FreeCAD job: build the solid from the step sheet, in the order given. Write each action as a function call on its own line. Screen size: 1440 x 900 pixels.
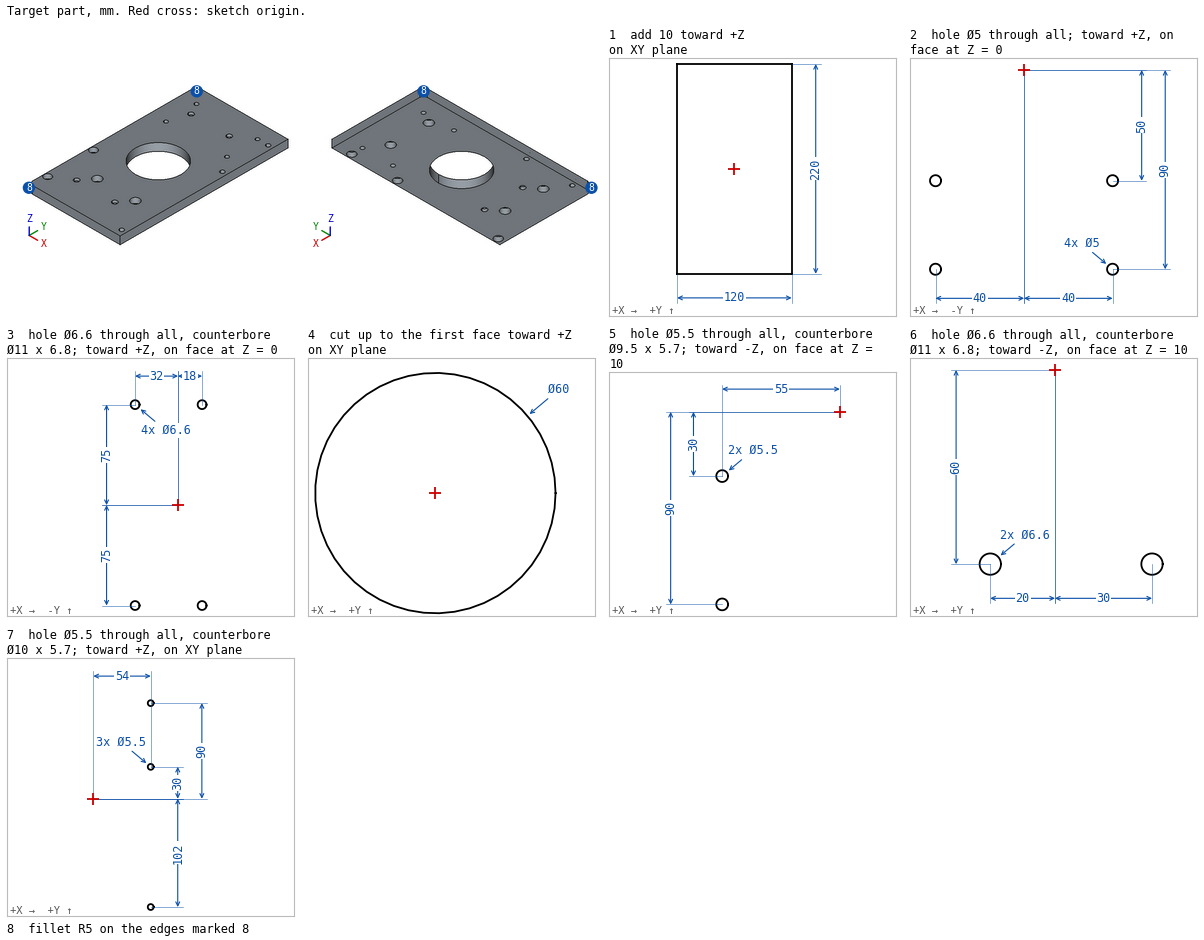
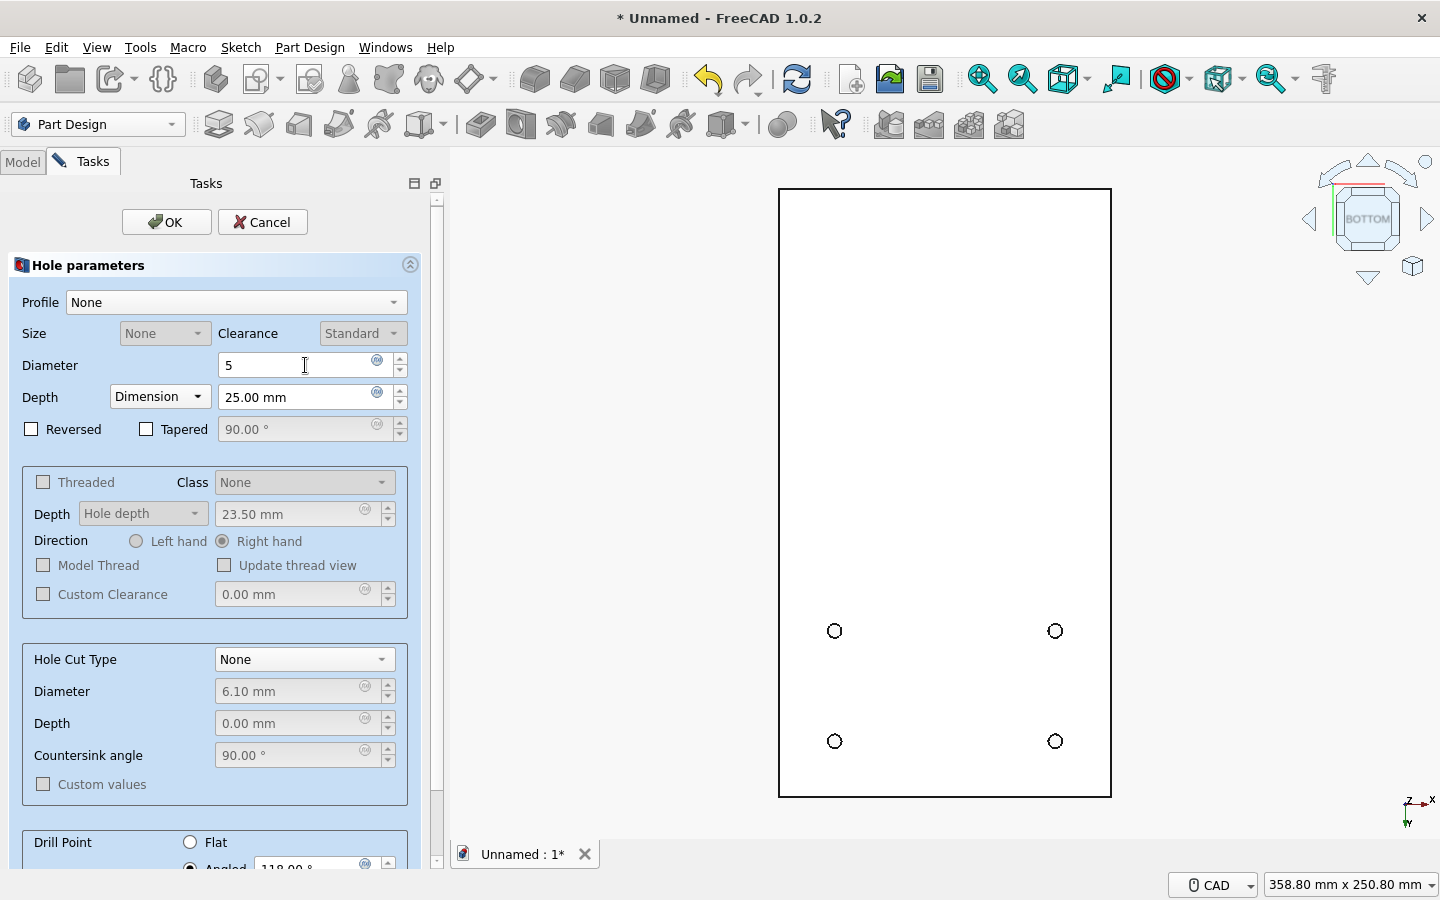
click(161, 396)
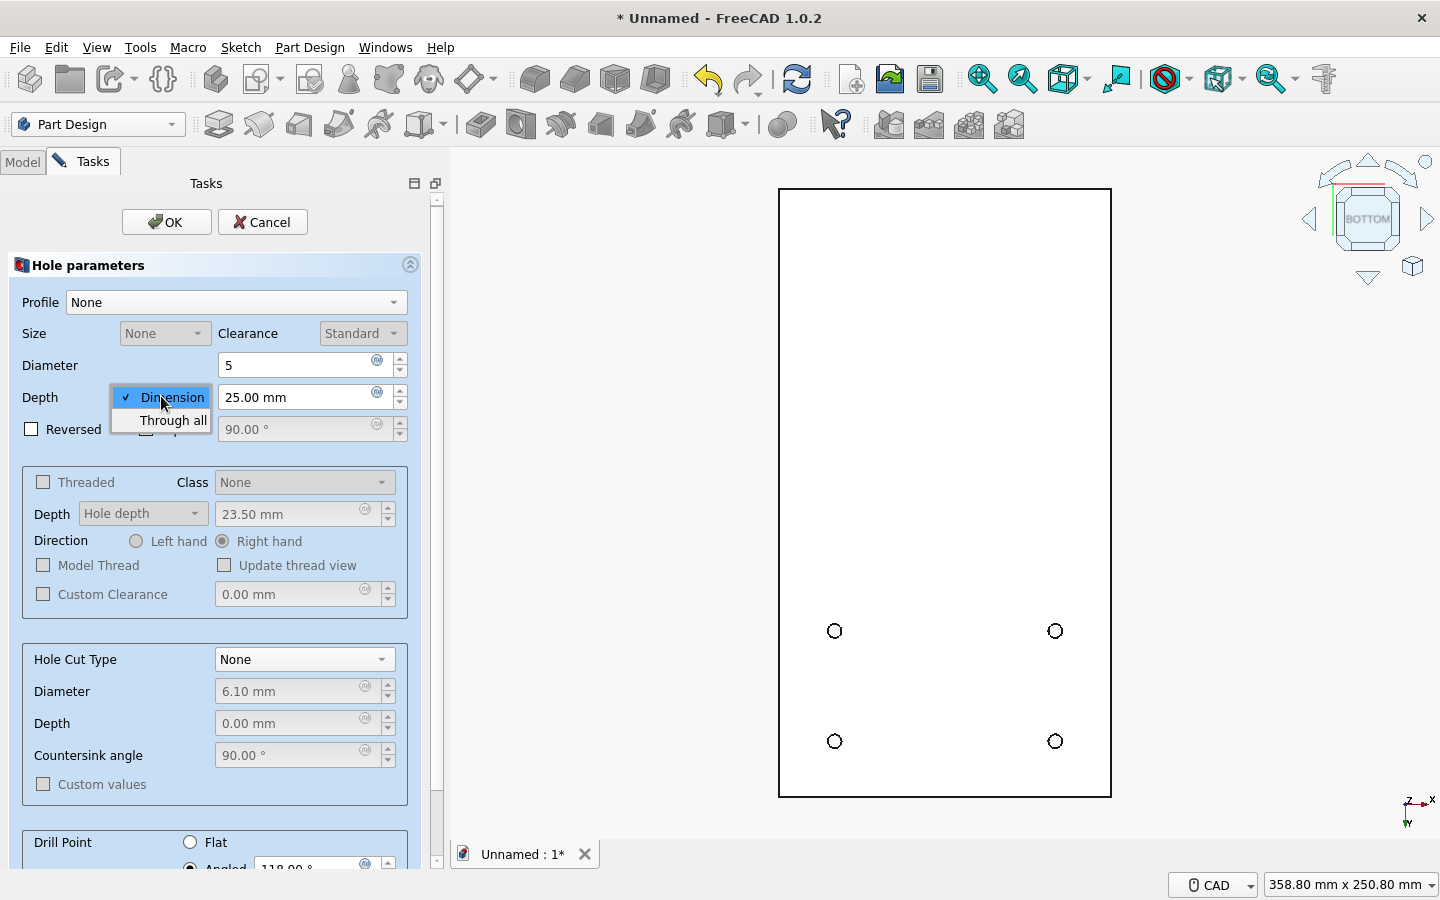
click(160, 420)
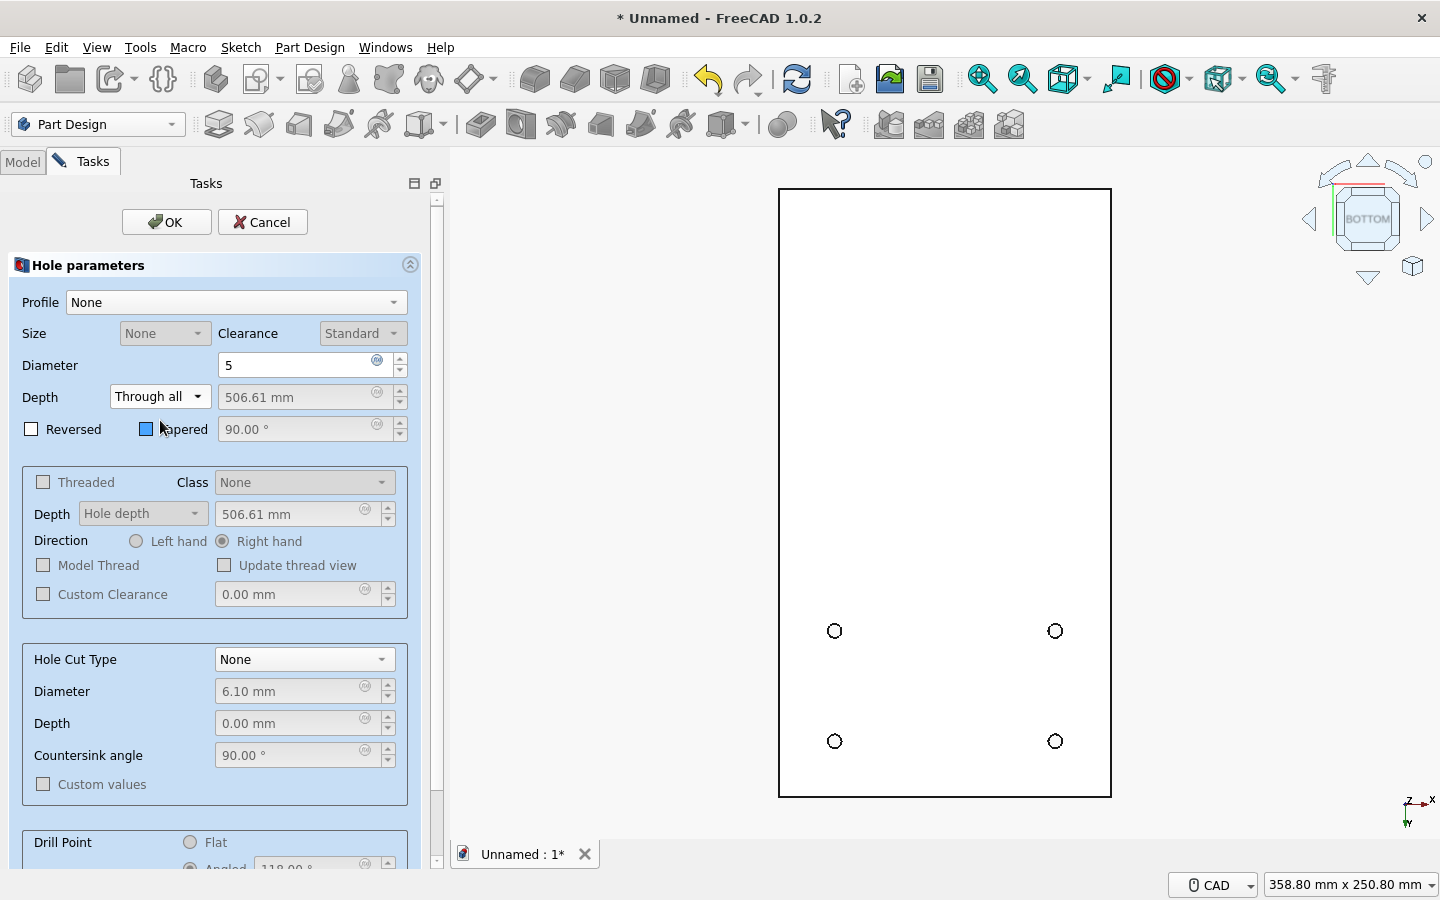
click(167, 222)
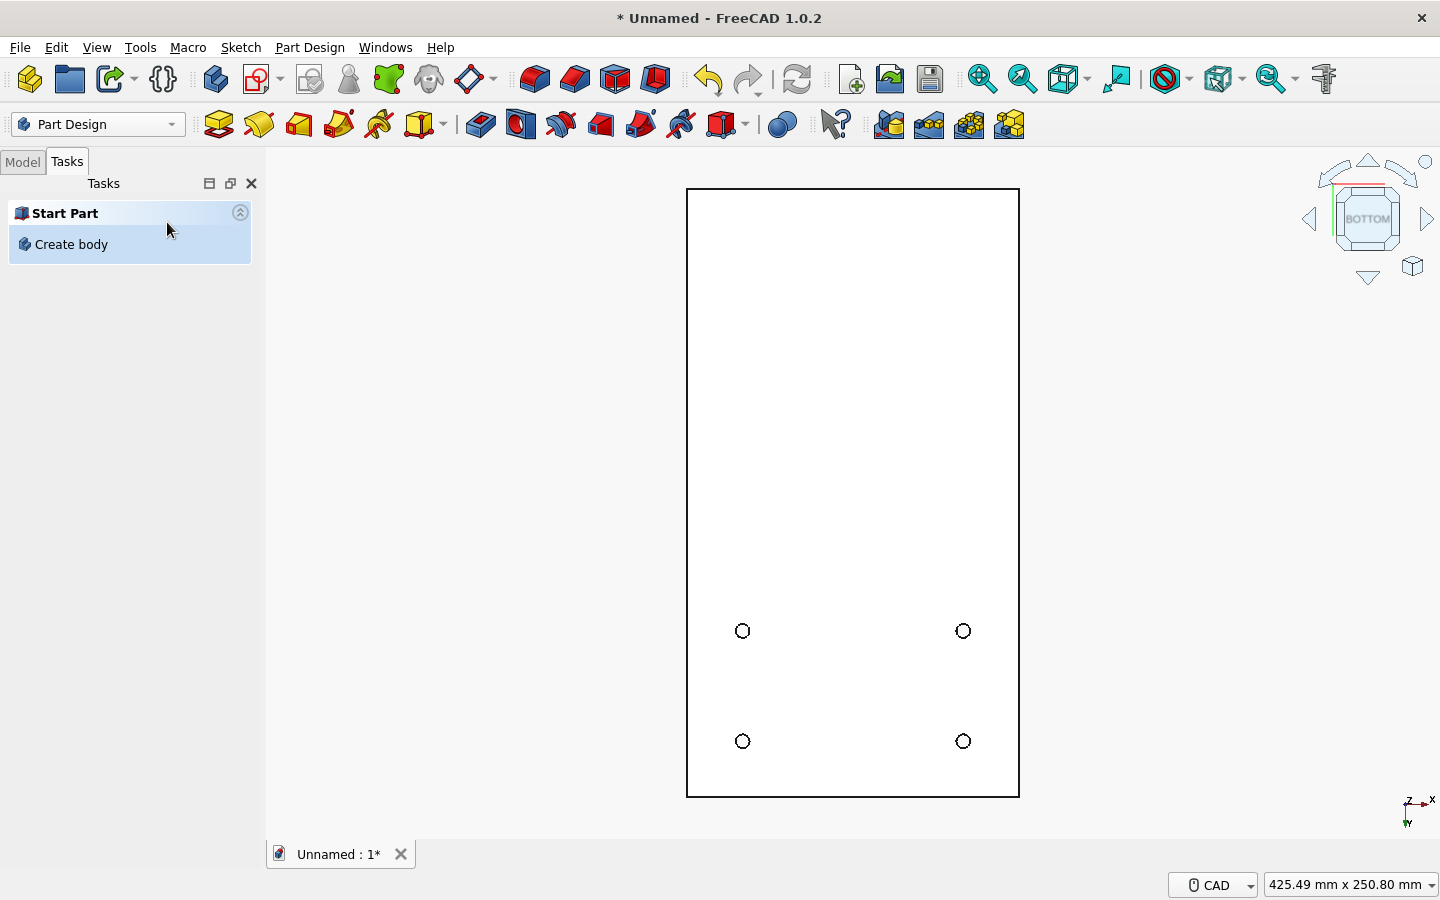
click(853, 492)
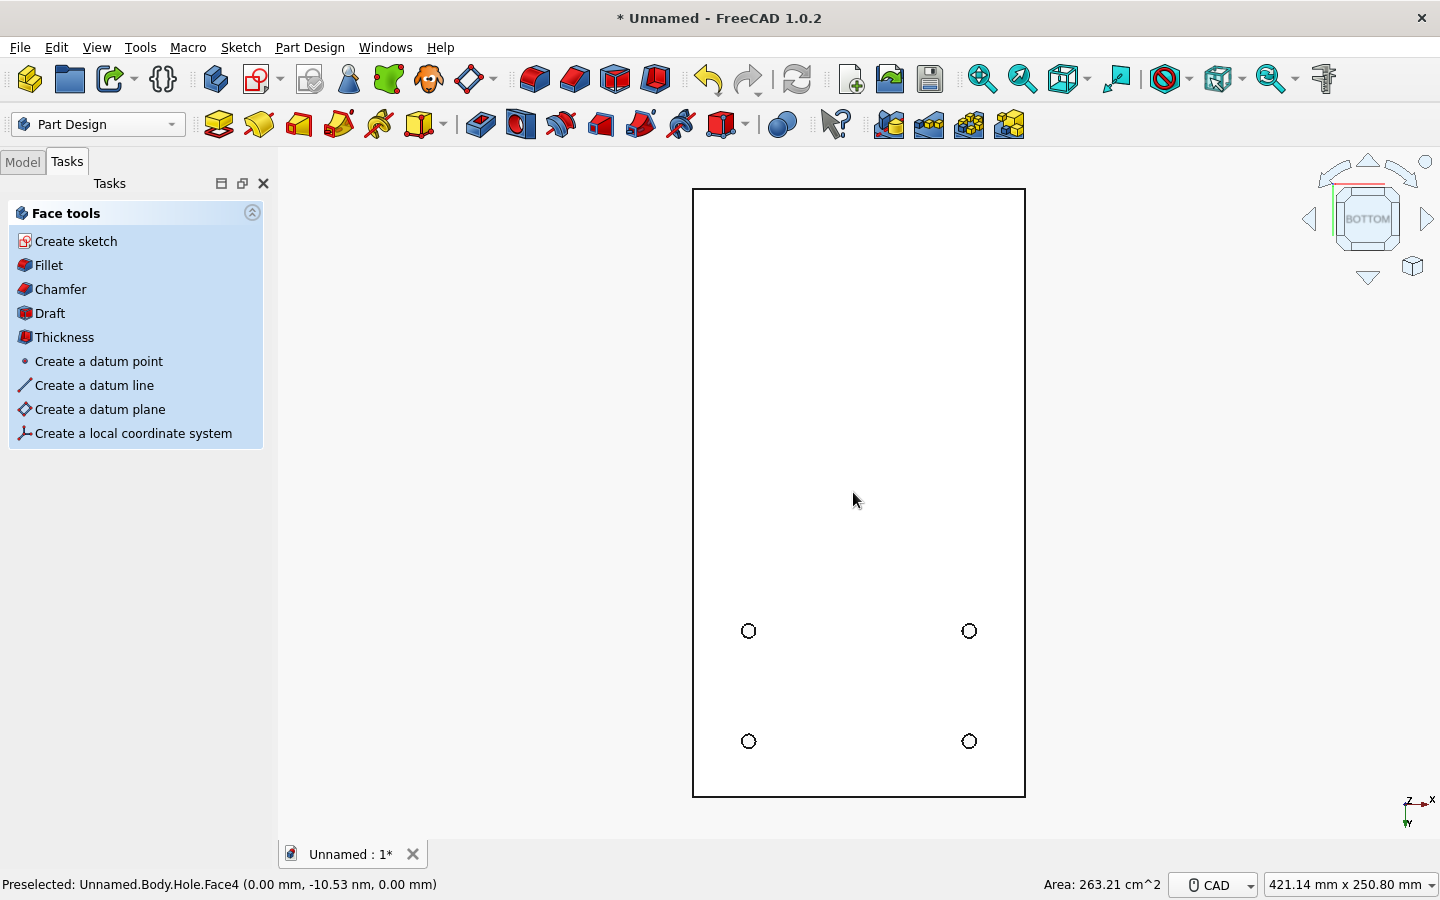
click(256, 80)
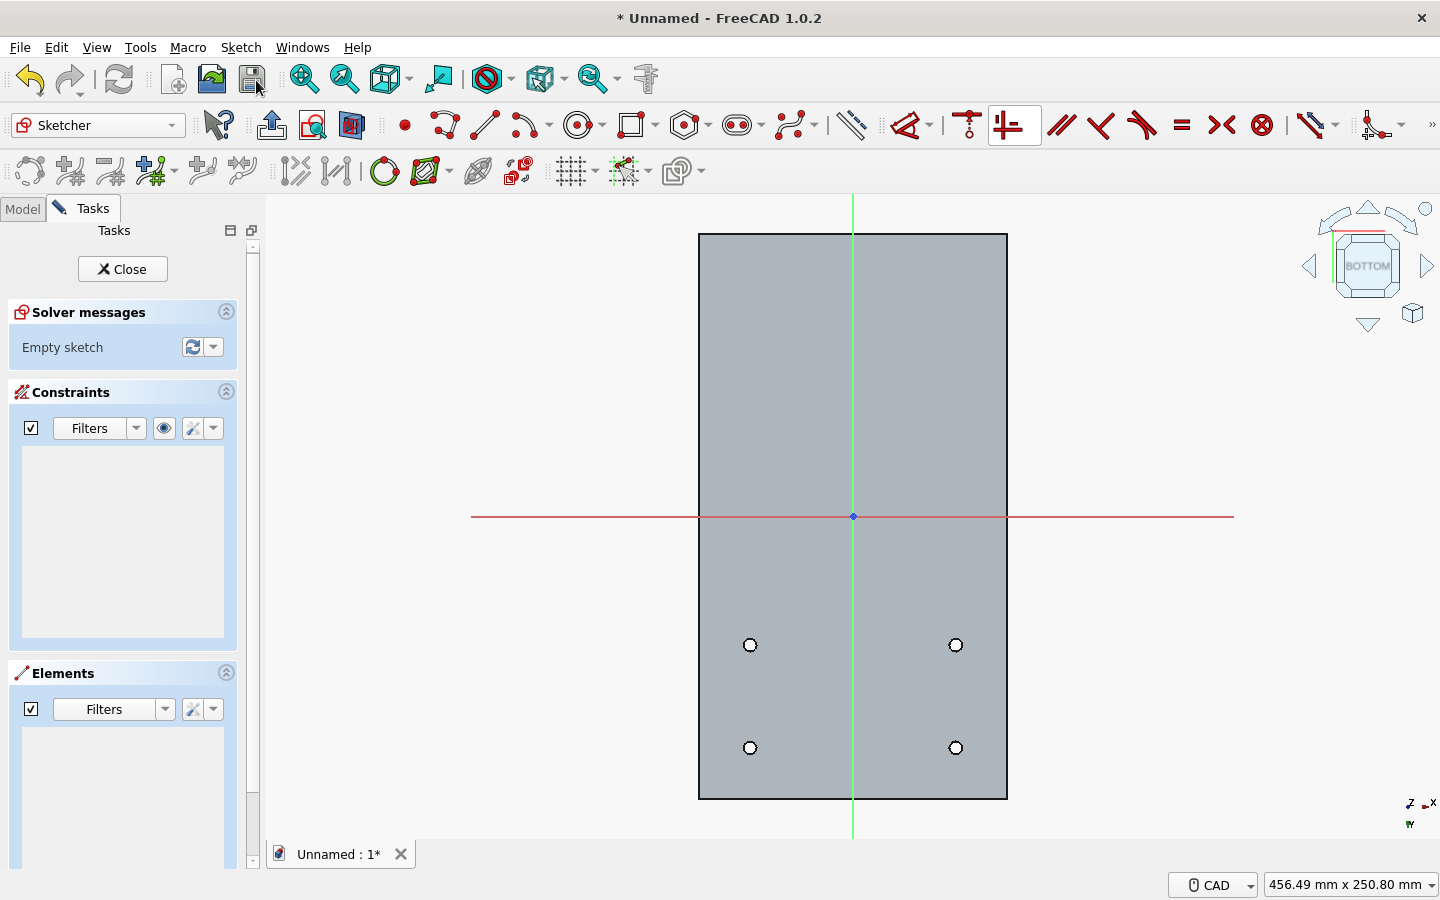
key(g)
key(c)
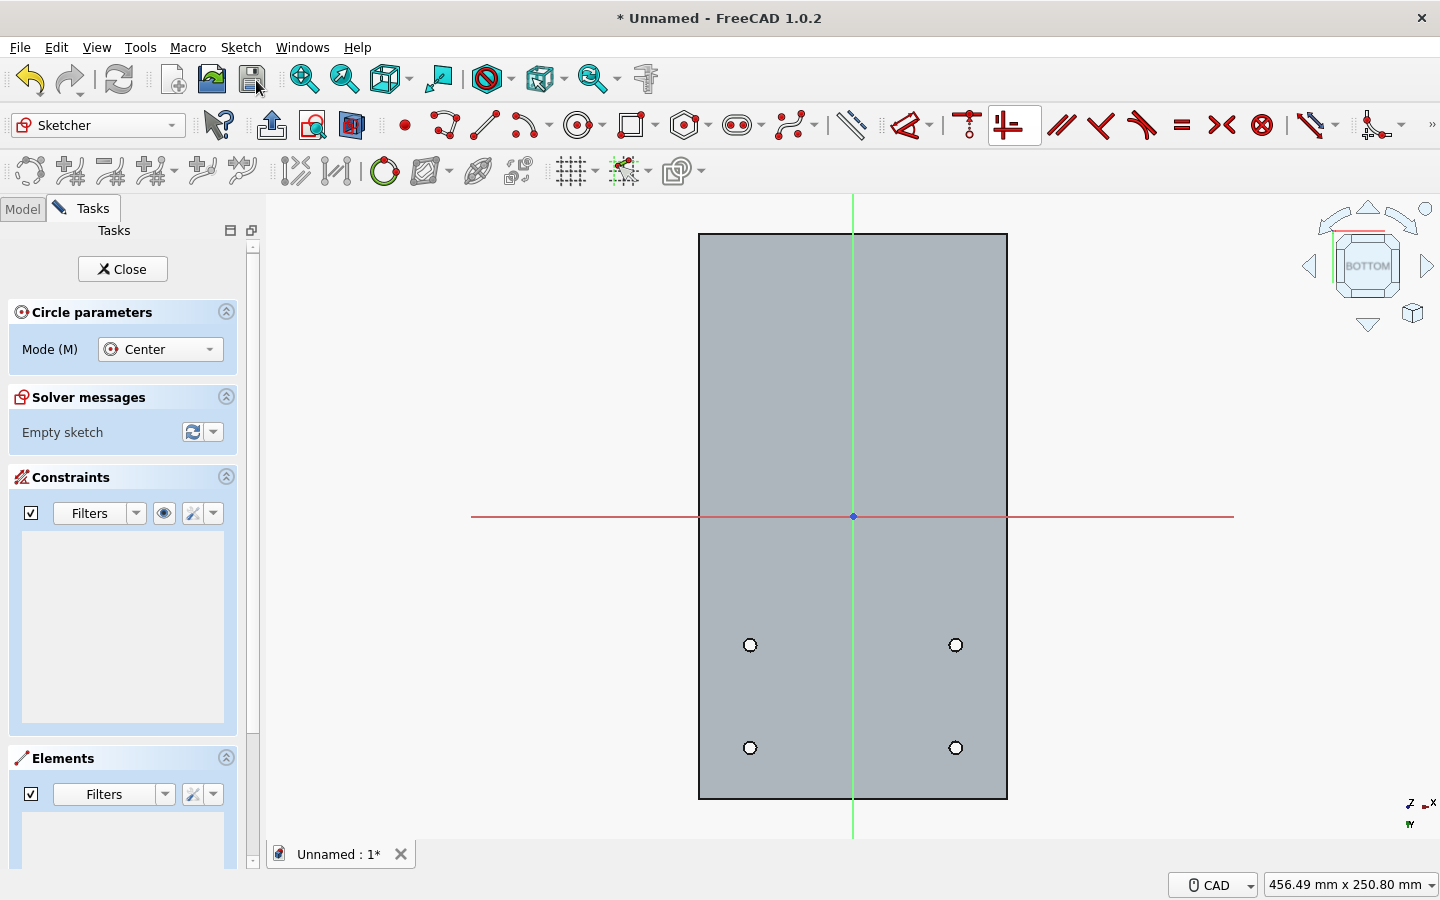
scroll(771, 324, up, 5)